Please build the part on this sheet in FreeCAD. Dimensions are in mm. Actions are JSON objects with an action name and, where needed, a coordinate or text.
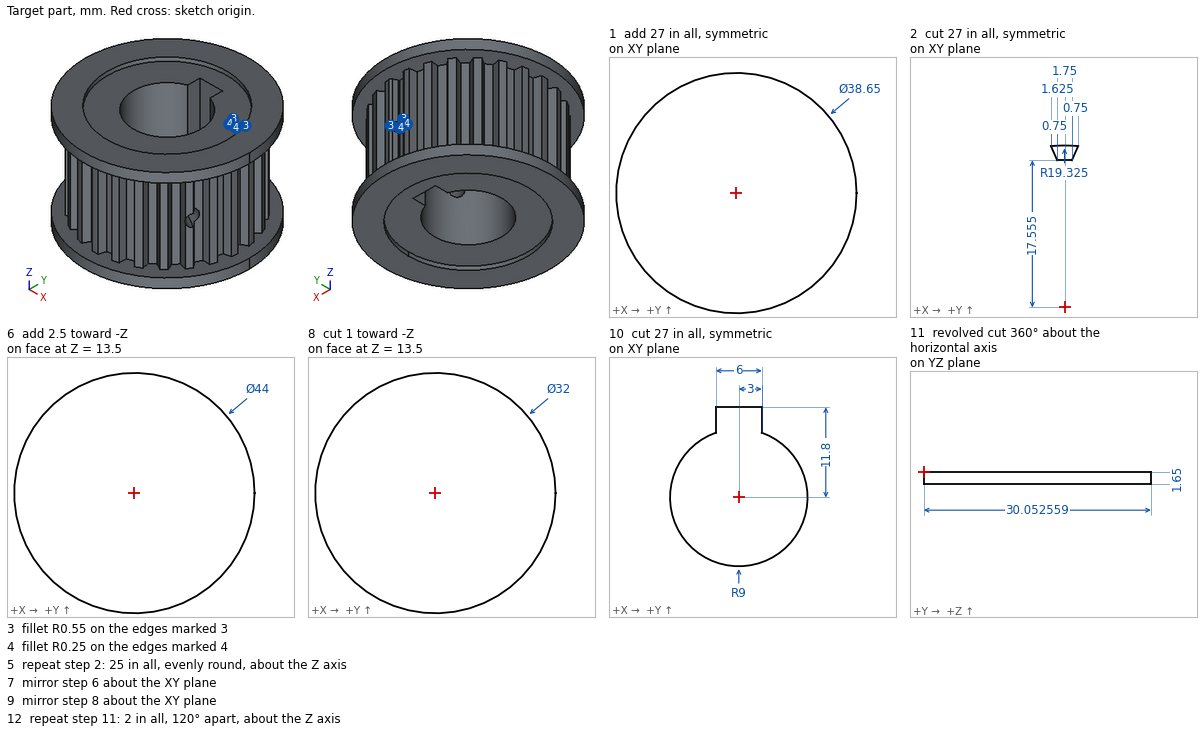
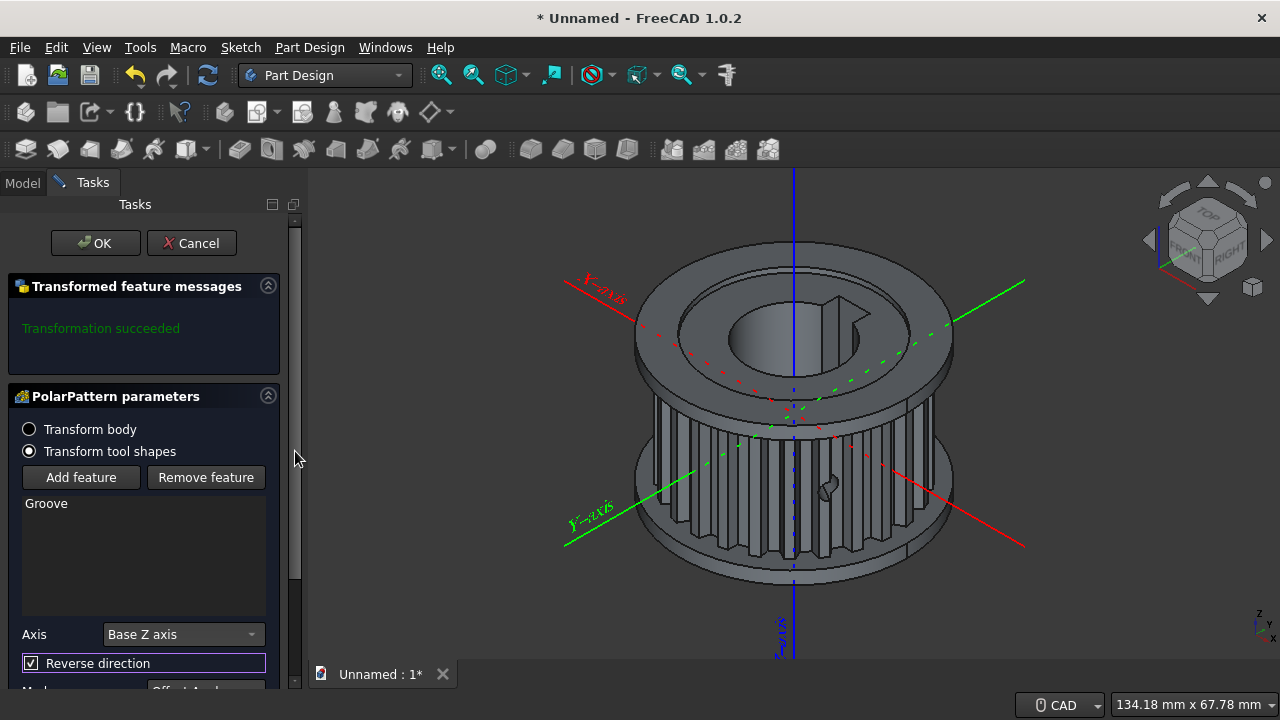
{"action": "left_click", "coordinate": [96, 243]}